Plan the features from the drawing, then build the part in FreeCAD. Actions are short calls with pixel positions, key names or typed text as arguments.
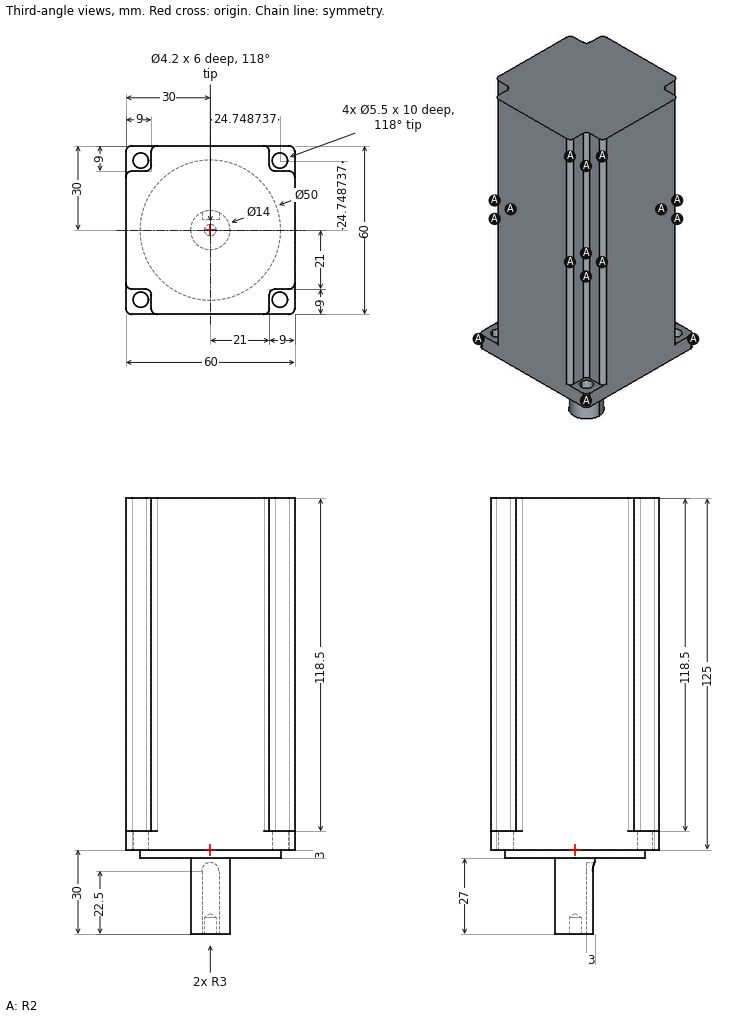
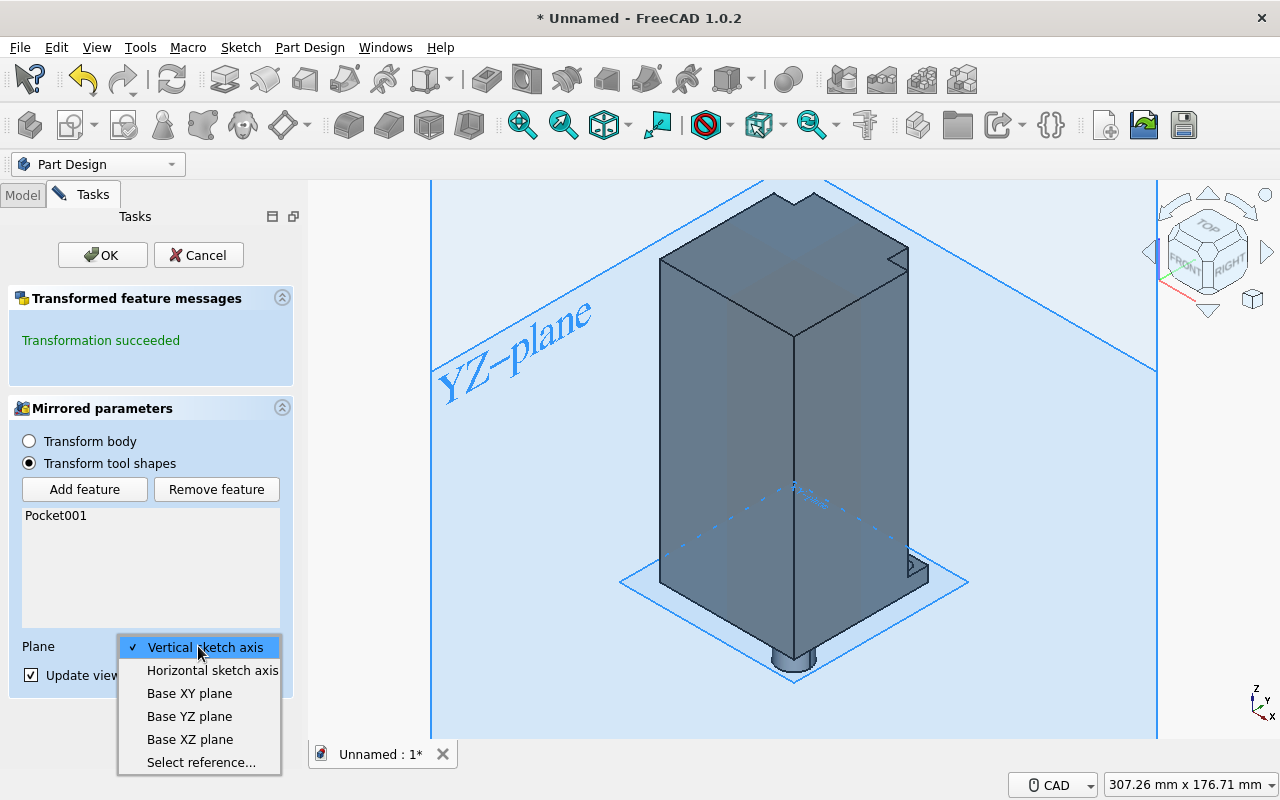
click(198, 716)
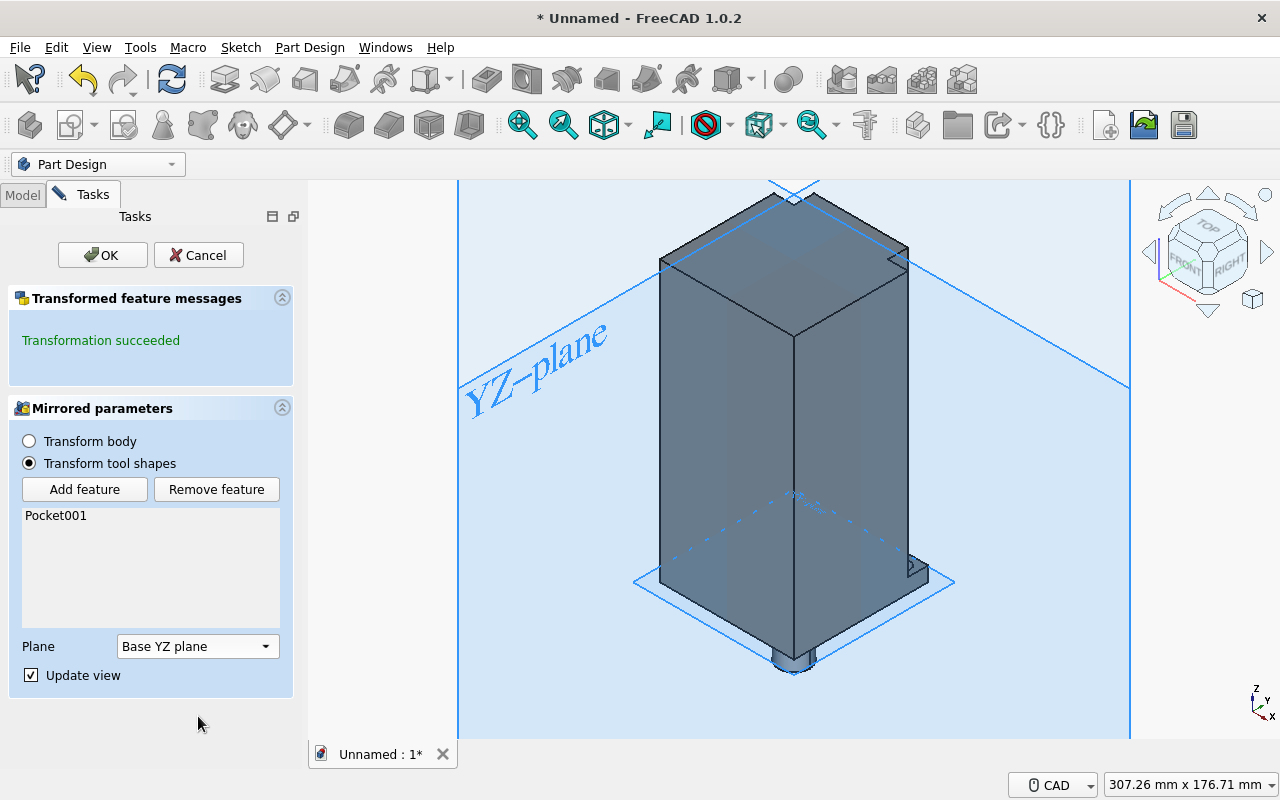
click(103, 255)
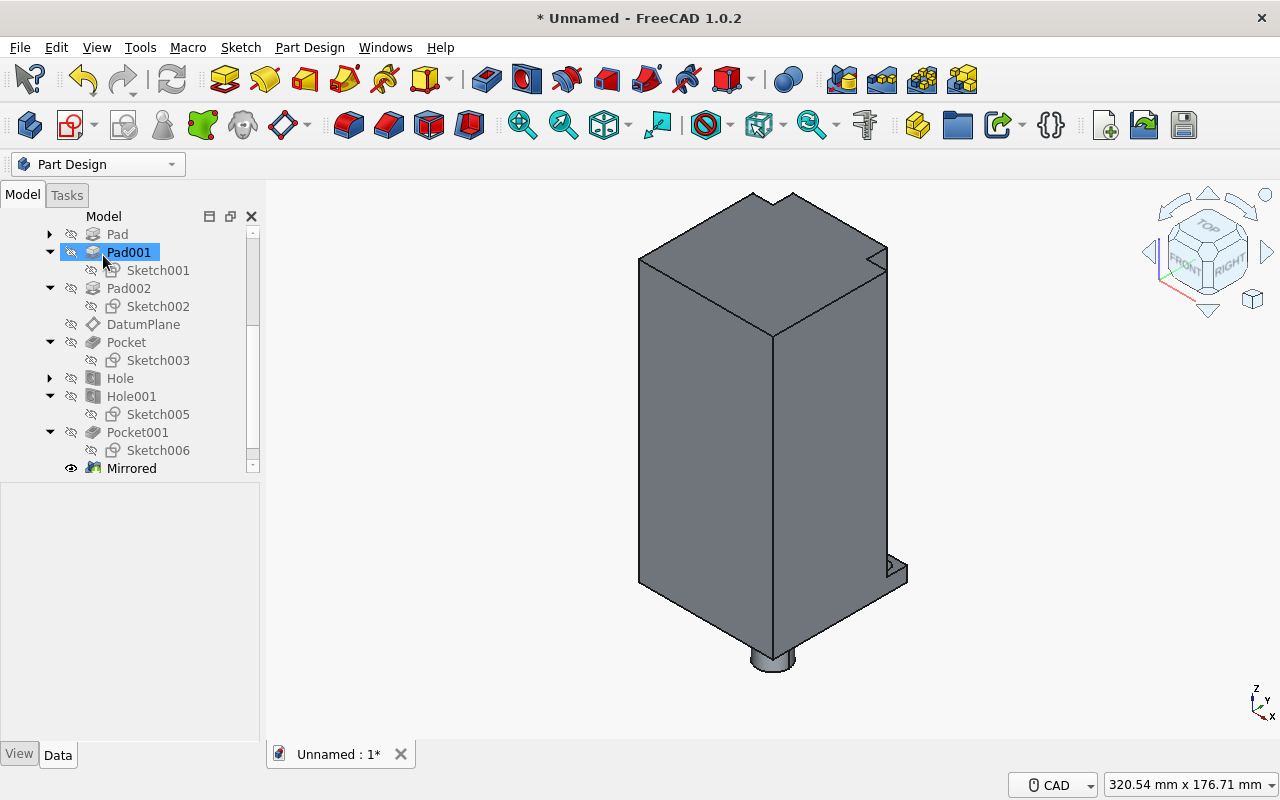
click(116, 432)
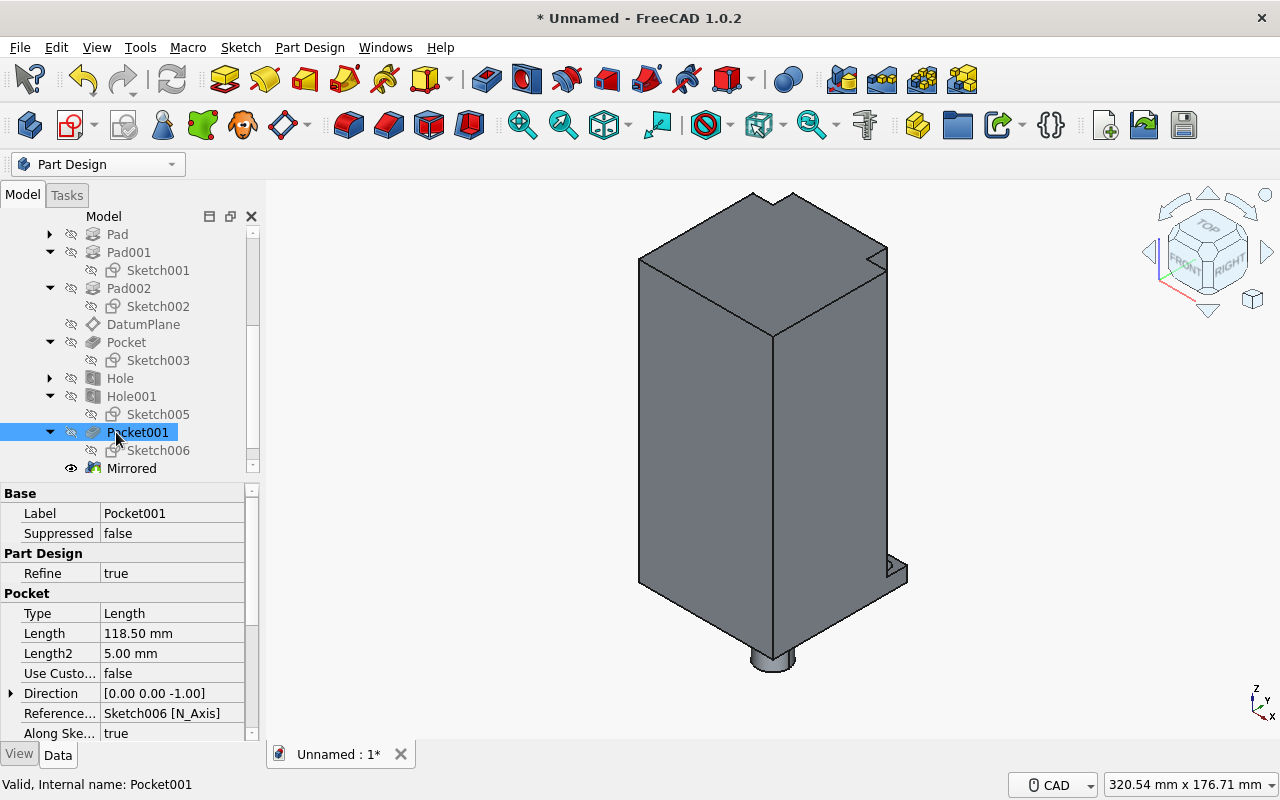
click(842, 80)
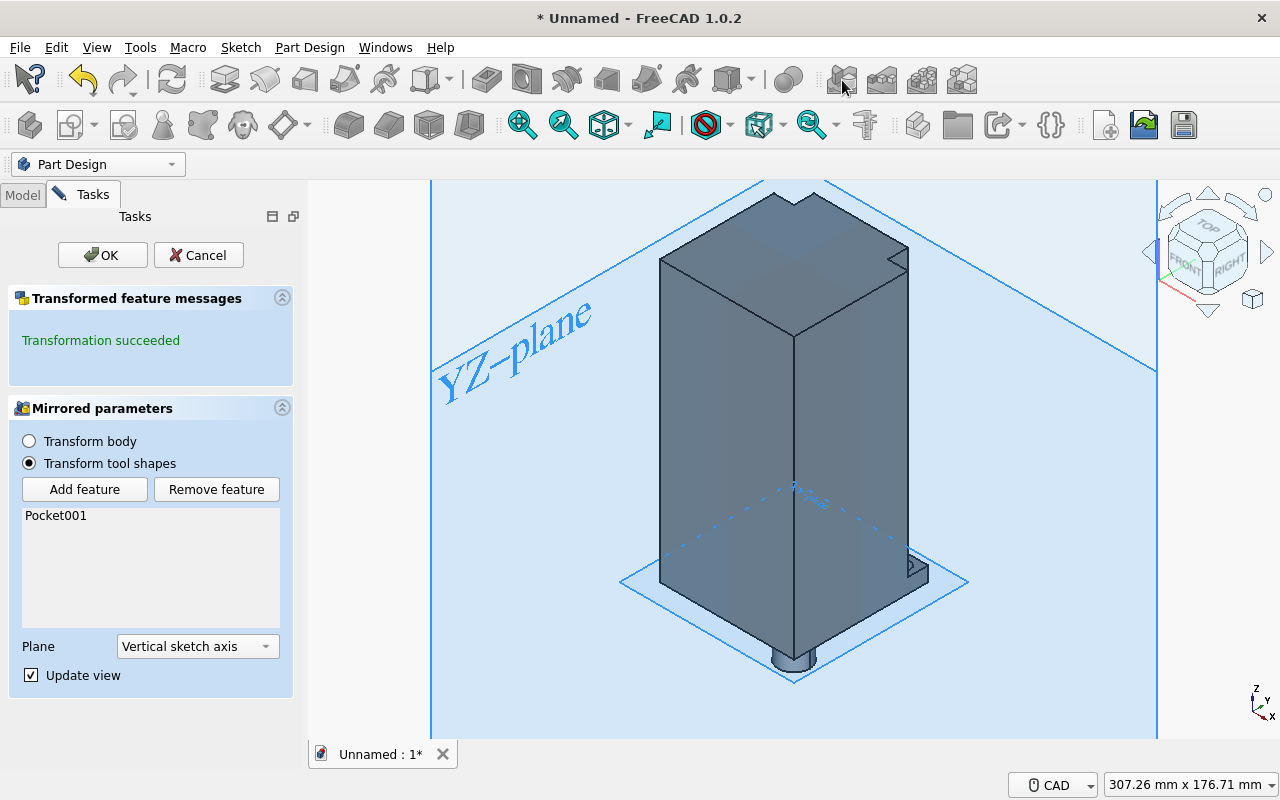
click(198, 646)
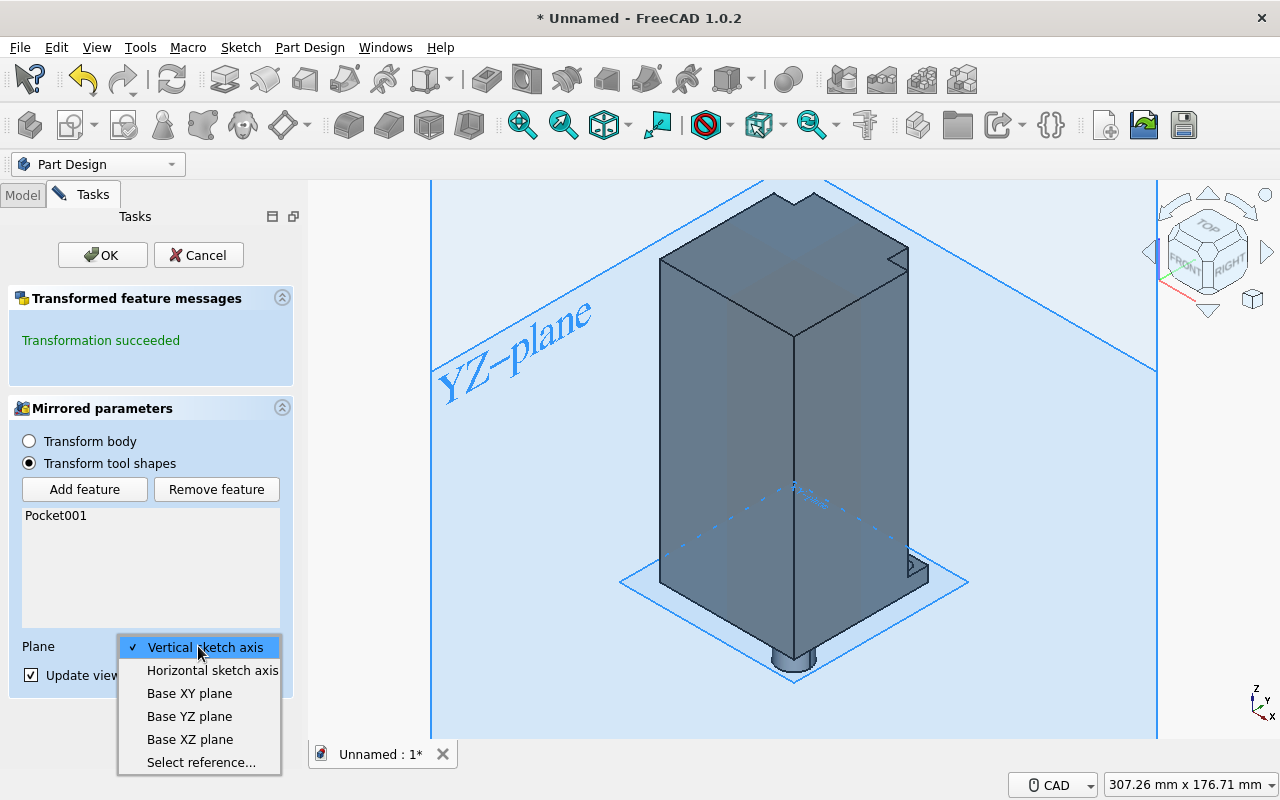
click(198, 740)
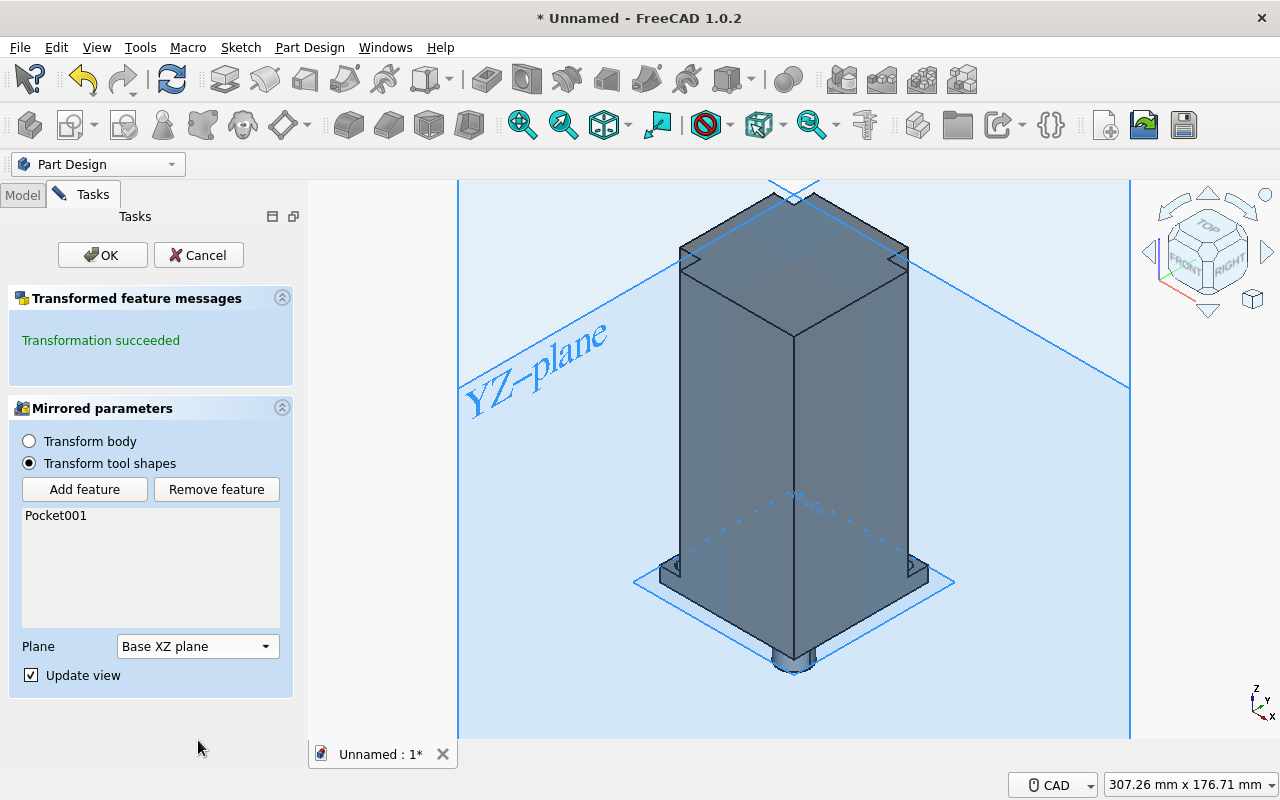
click(103, 255)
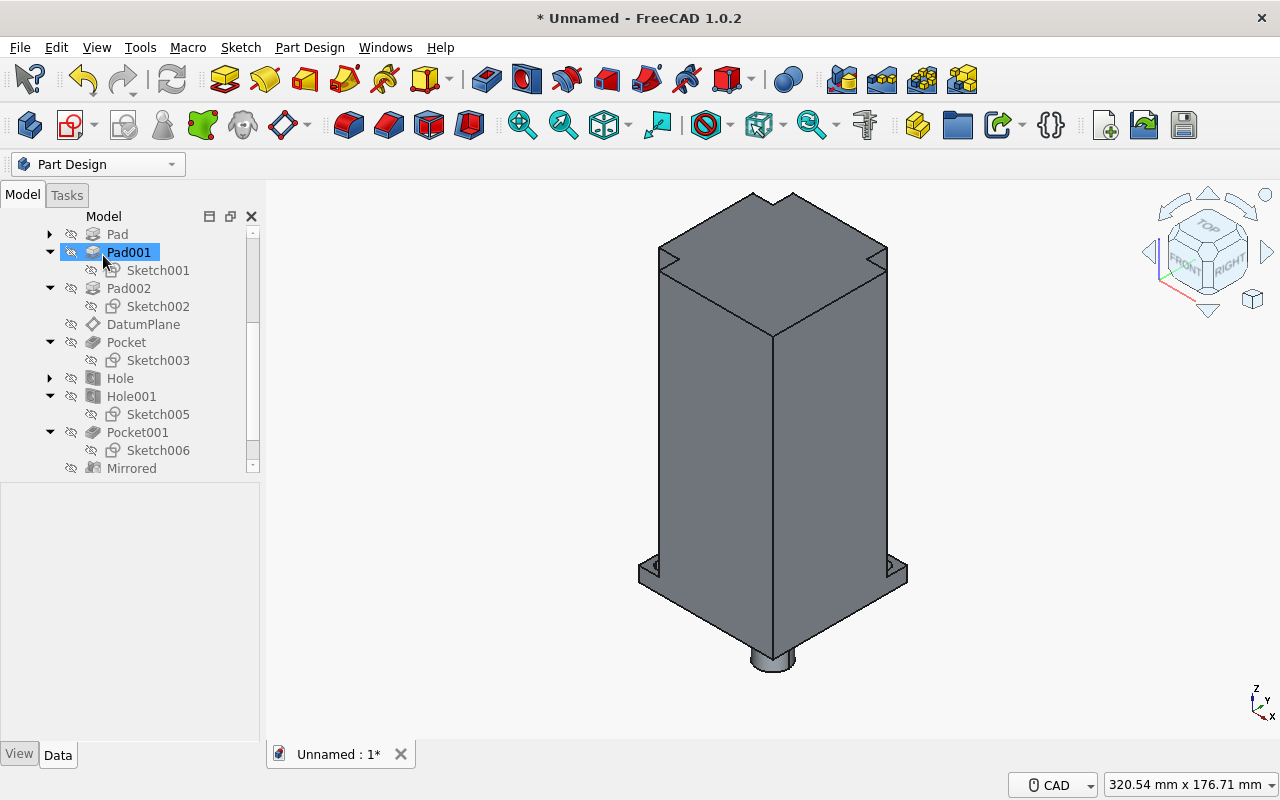
click(773, 258)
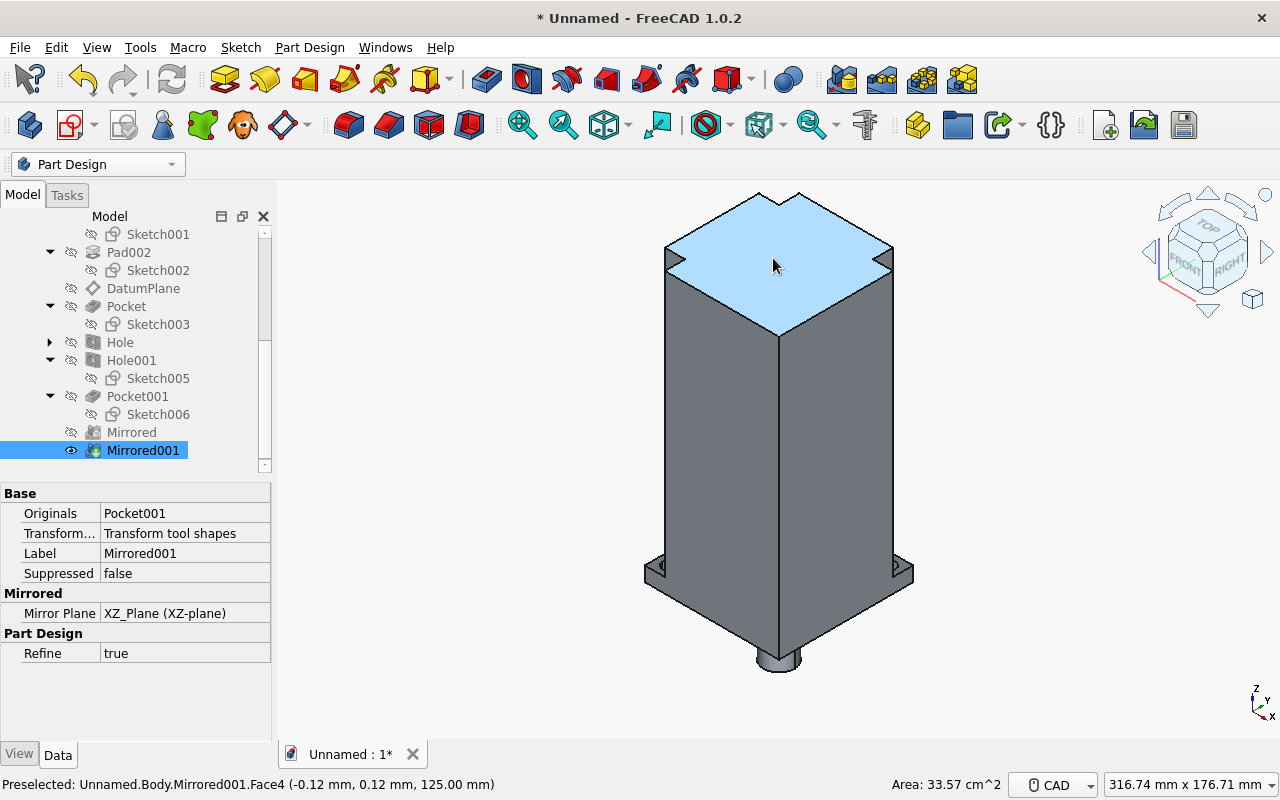
click(70, 126)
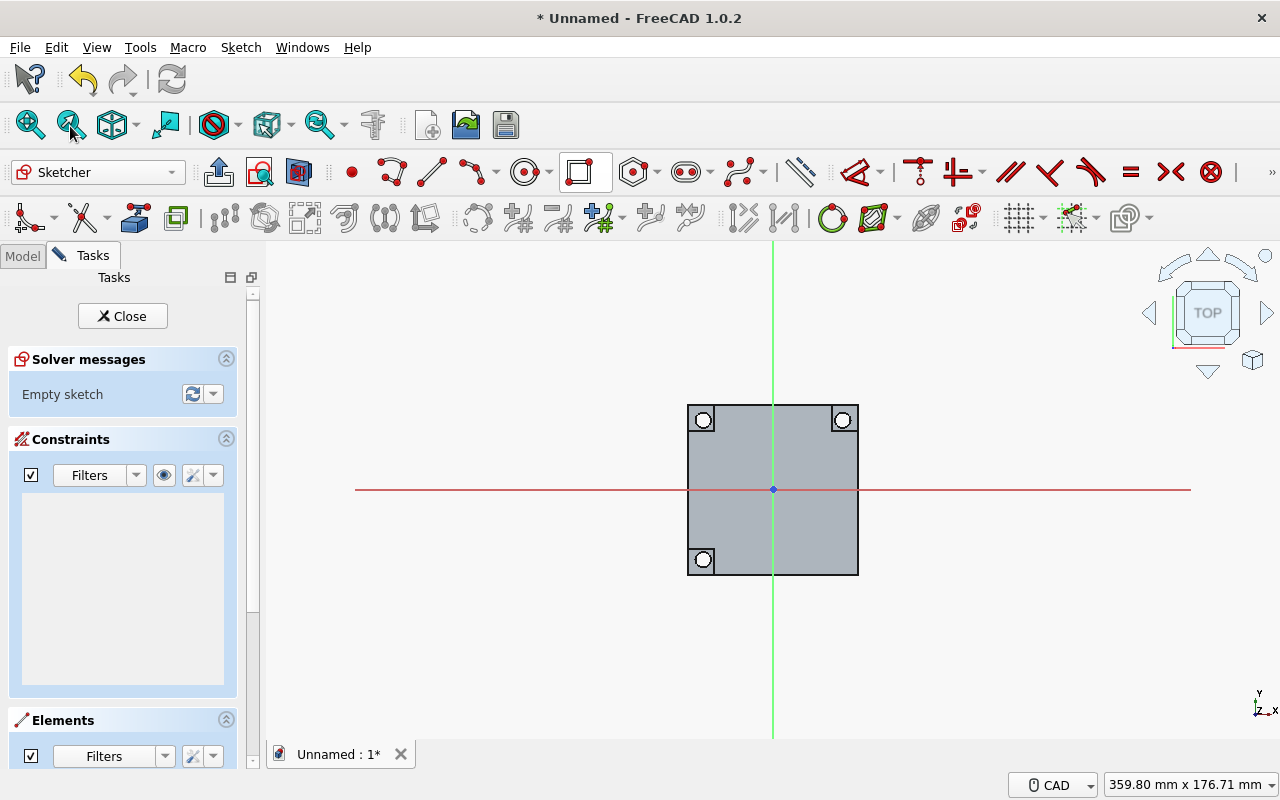
scroll(856, 568, up, 13)